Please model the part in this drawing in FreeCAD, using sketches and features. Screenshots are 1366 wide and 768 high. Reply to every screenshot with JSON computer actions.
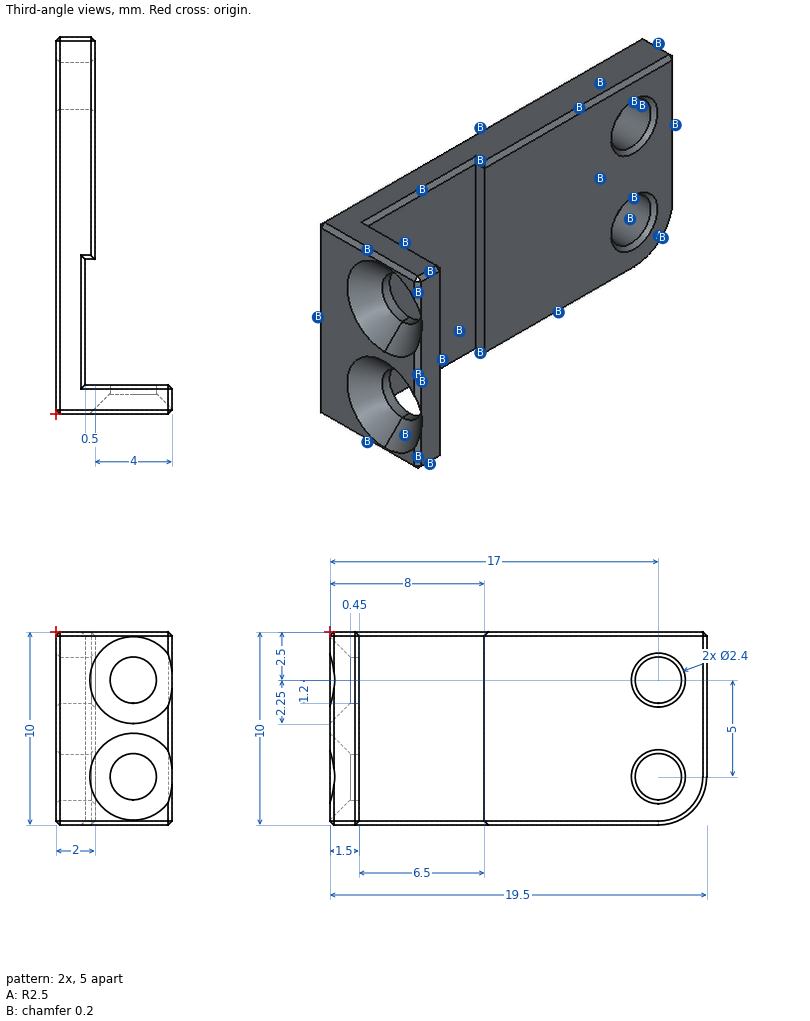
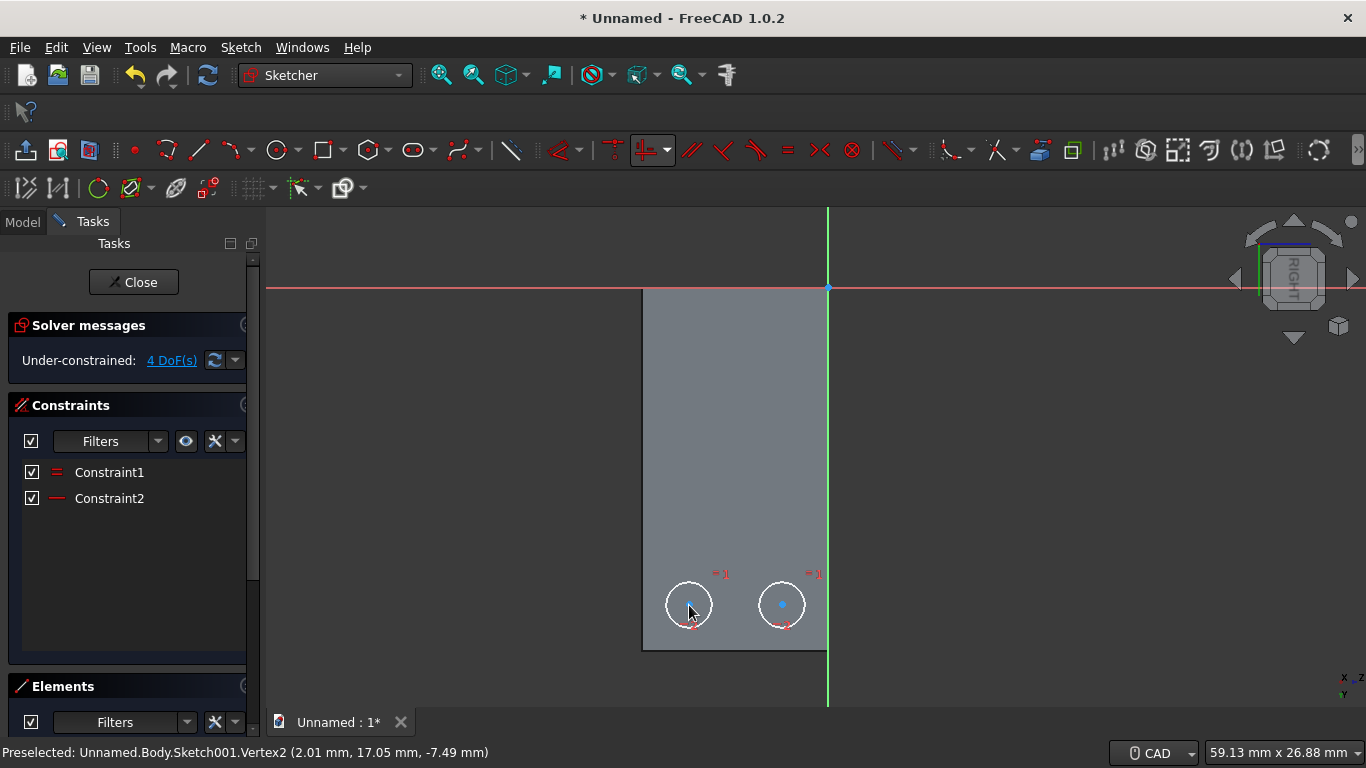
{"action": "left_click", "coordinate": [558, 150]}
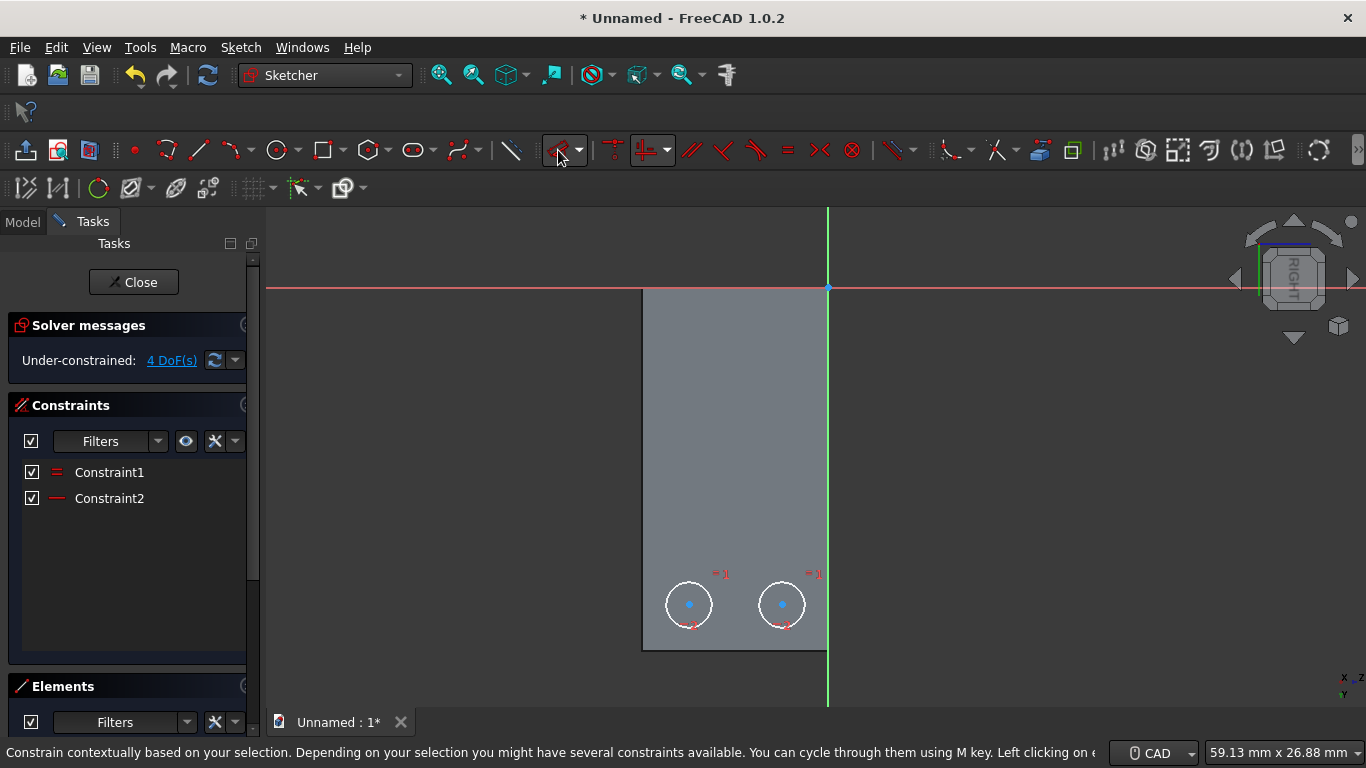
{"action": "left_click", "coordinate": [798, 589]}
{"action": "left_click", "coordinate": [797, 553]}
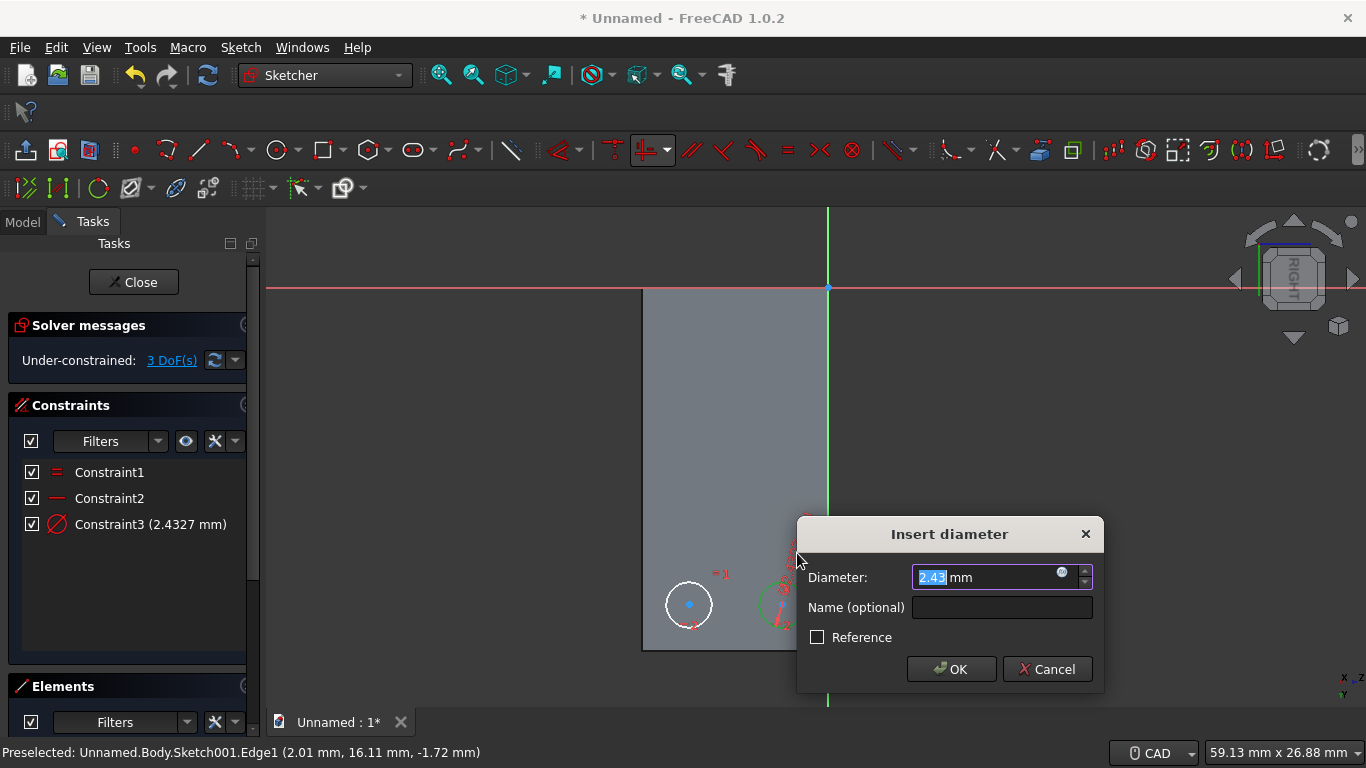
{"action": "type", "text": "2.4"}
{"action": "key", "text": "Return"}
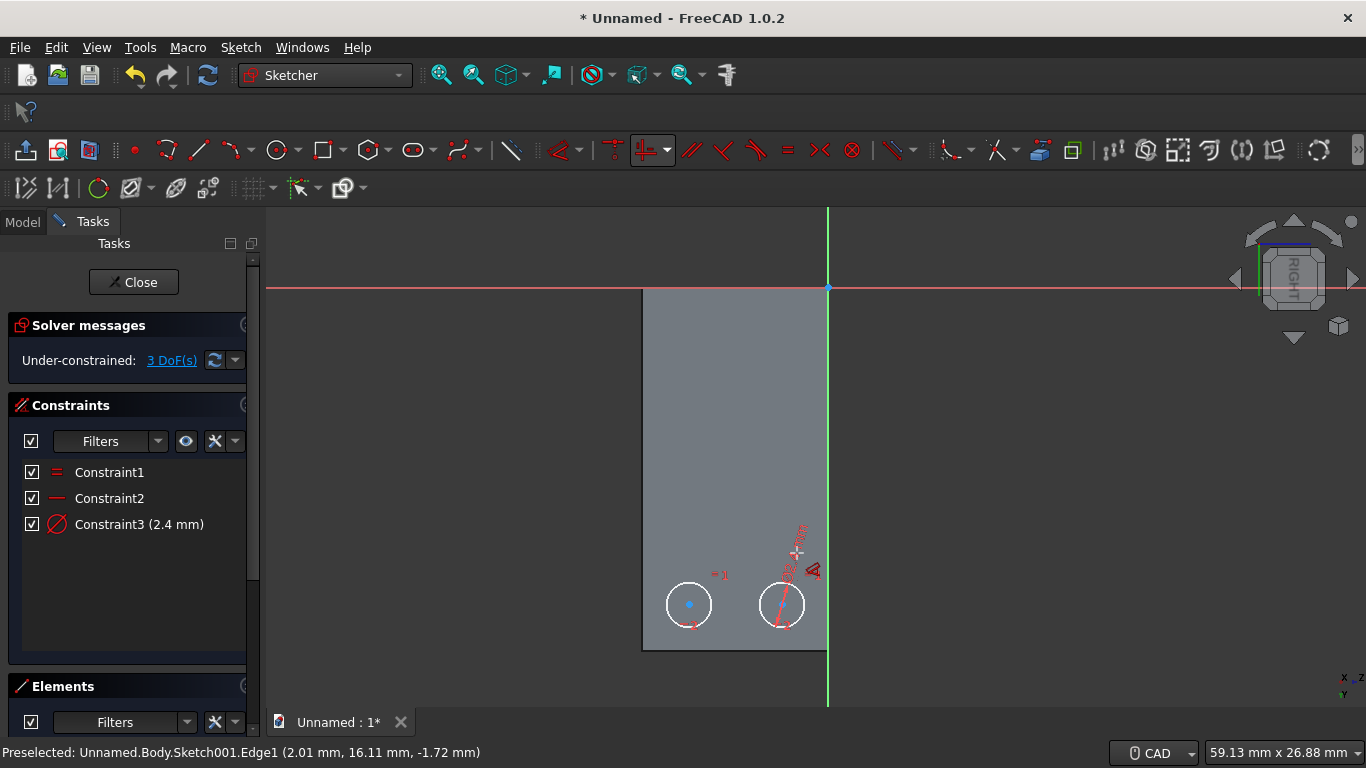
{"action": "left_click", "coordinate": [782, 605]}
{"action": "left_click", "coordinate": [862, 446]}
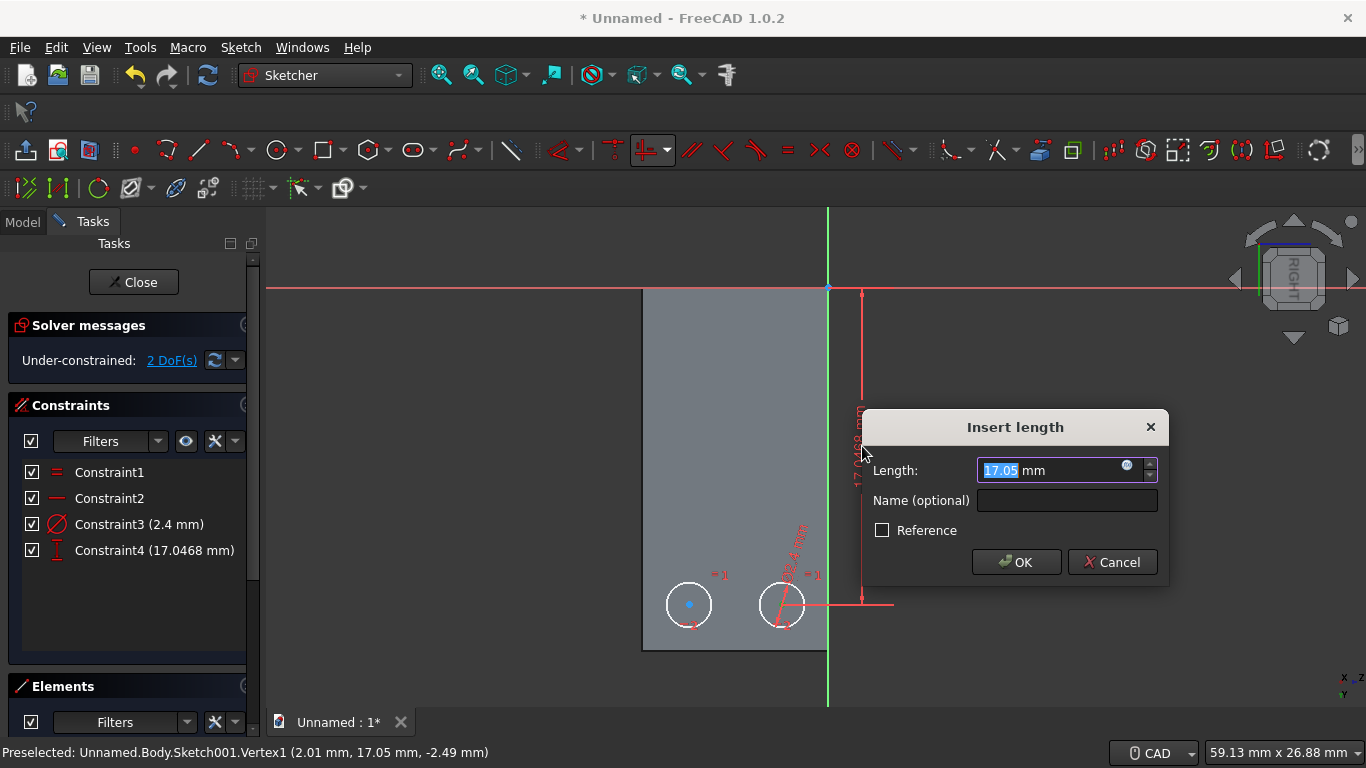
{"action": "type", "text": "17"}
{"action": "key", "text": "Return"}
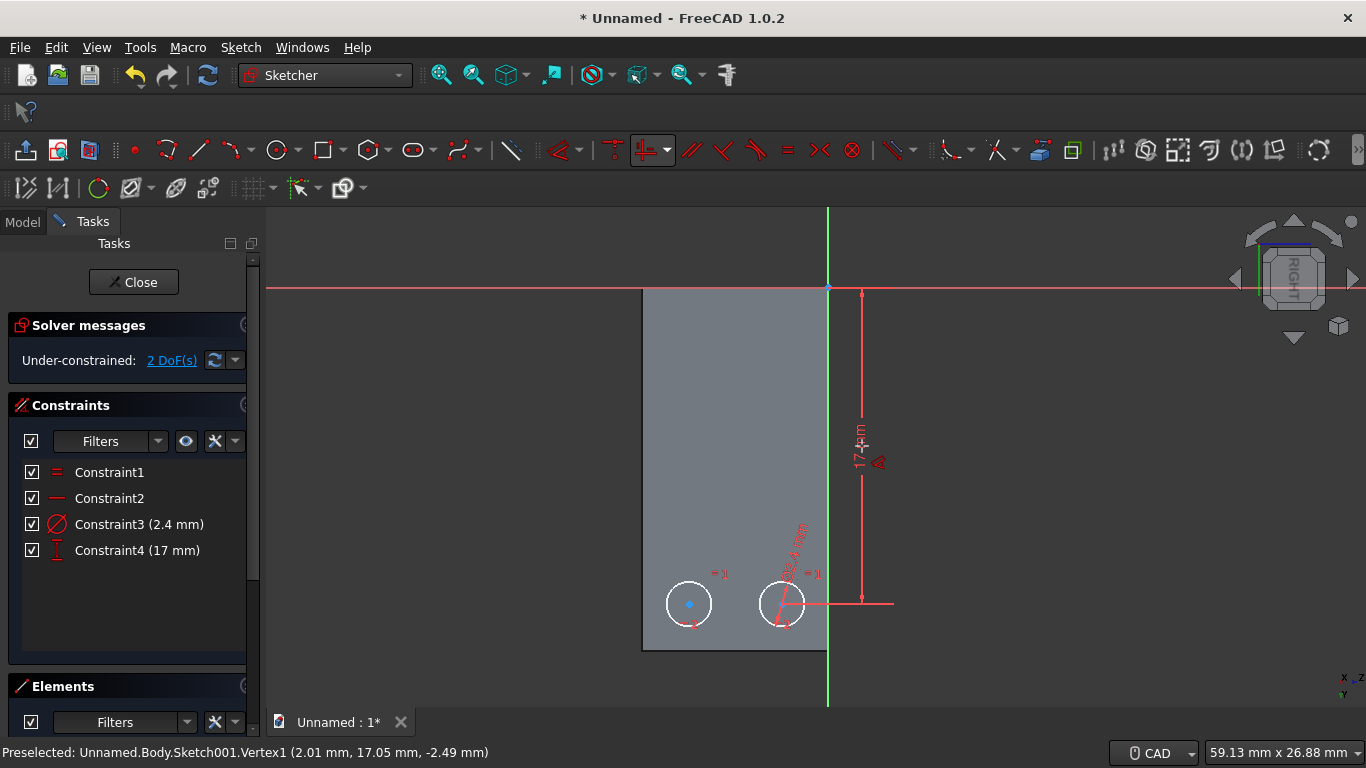
{"action": "left_click", "coordinate": [782, 604]}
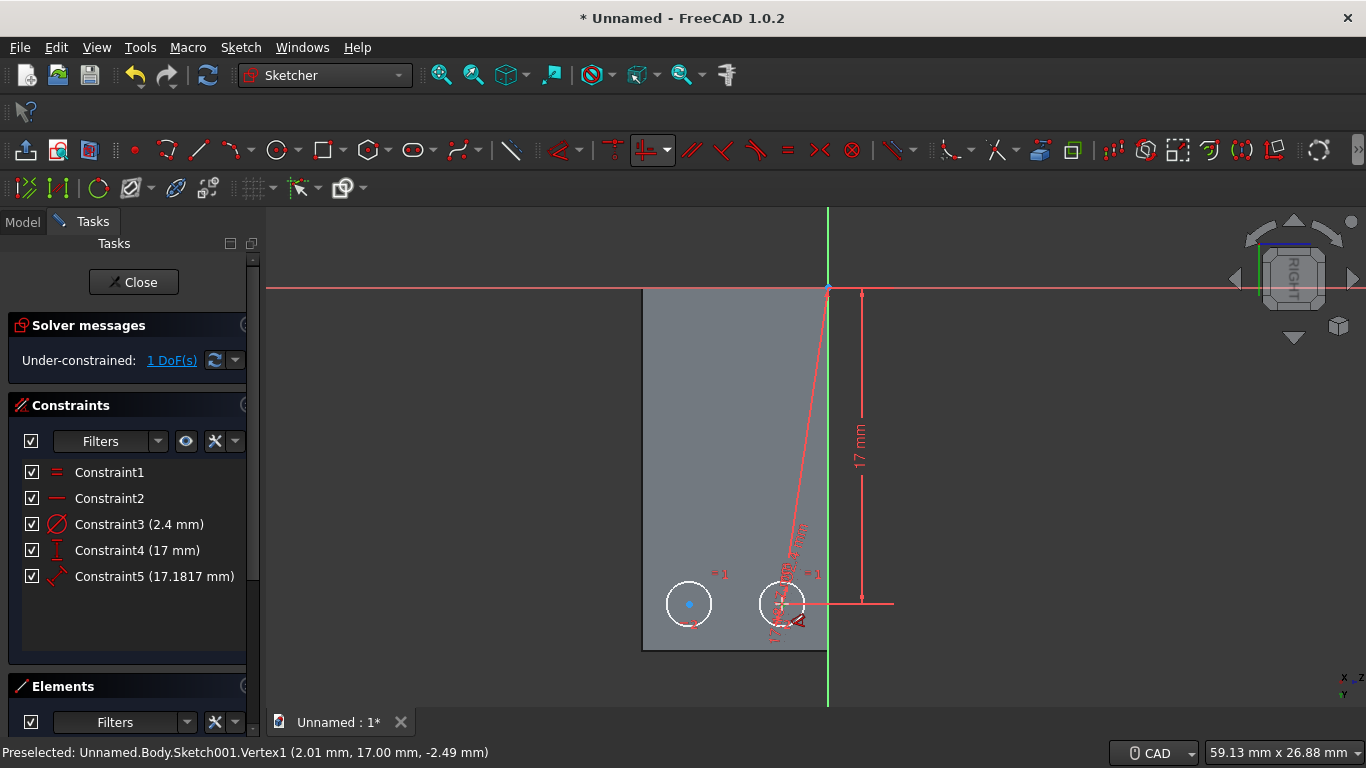
{"action": "left_click", "coordinate": [689, 604]}
{"action": "left_click", "coordinate": [735, 638]}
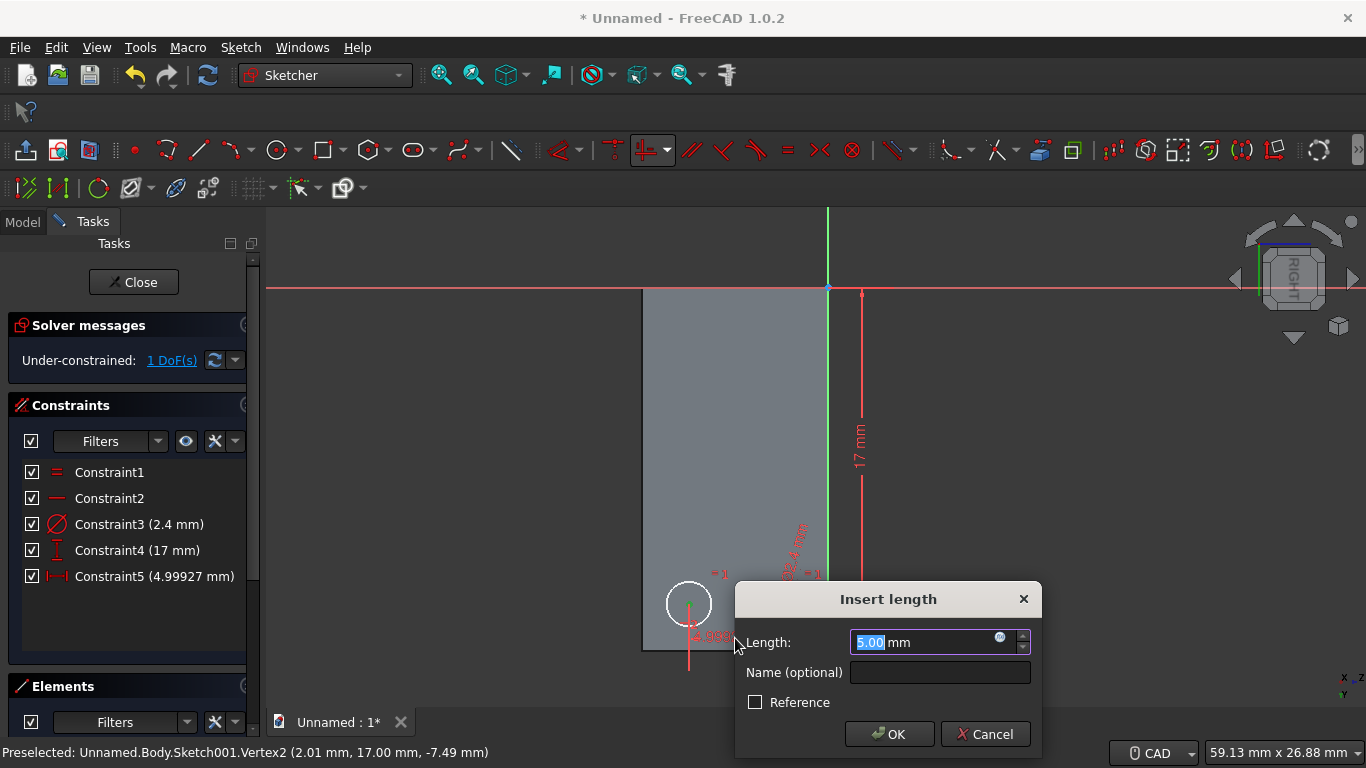
{"action": "type", "text": "5"}
{"action": "key", "text": "Return"}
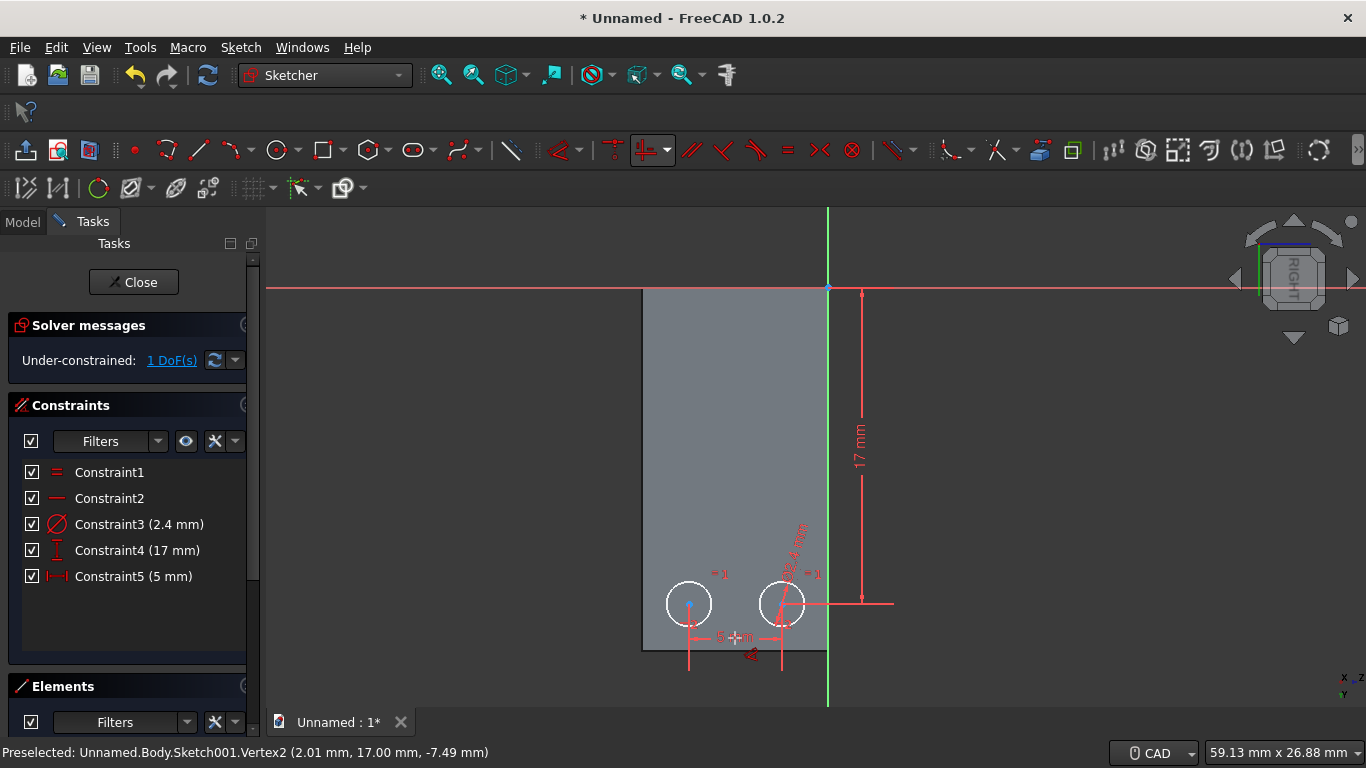
{"action": "left_click", "coordinate": [782, 604]}
{"action": "left_click", "coordinate": [805, 254]}